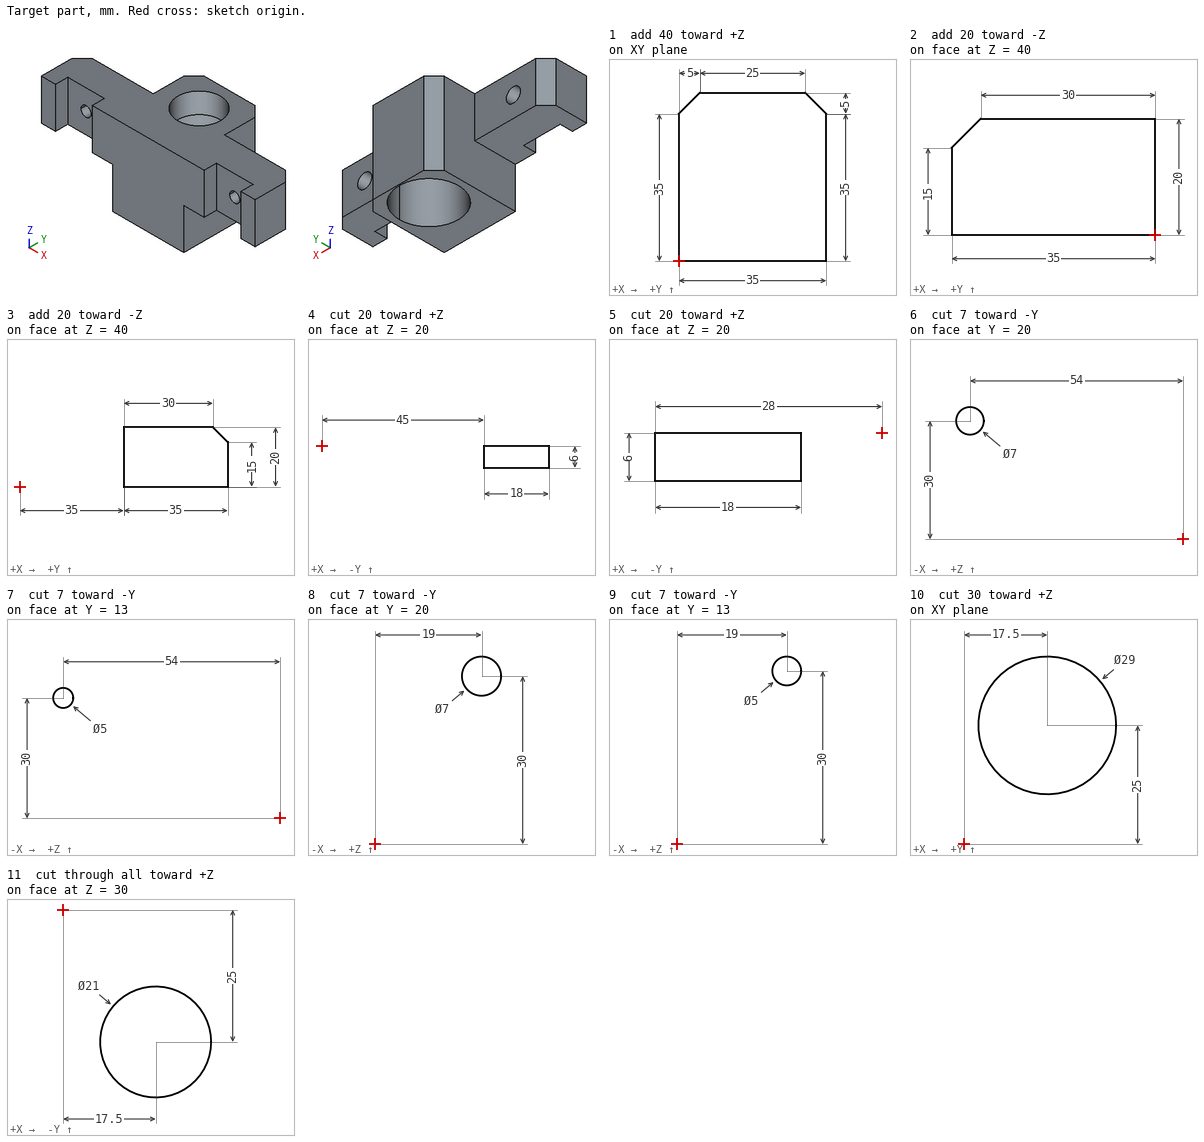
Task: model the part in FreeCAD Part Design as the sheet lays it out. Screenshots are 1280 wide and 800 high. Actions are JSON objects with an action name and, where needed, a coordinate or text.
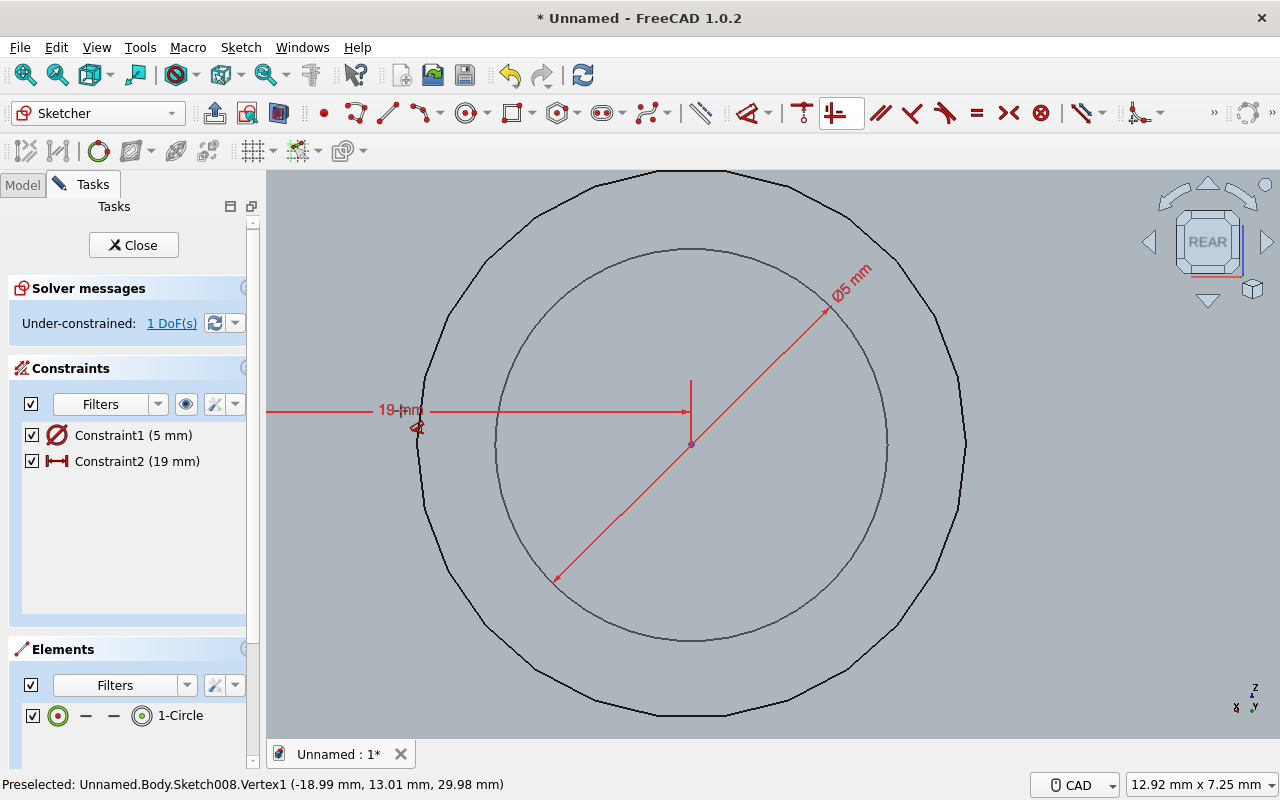
{"action": "left_click", "coordinate": [691, 445]}
{"action": "left_click", "coordinate": [725, 578]}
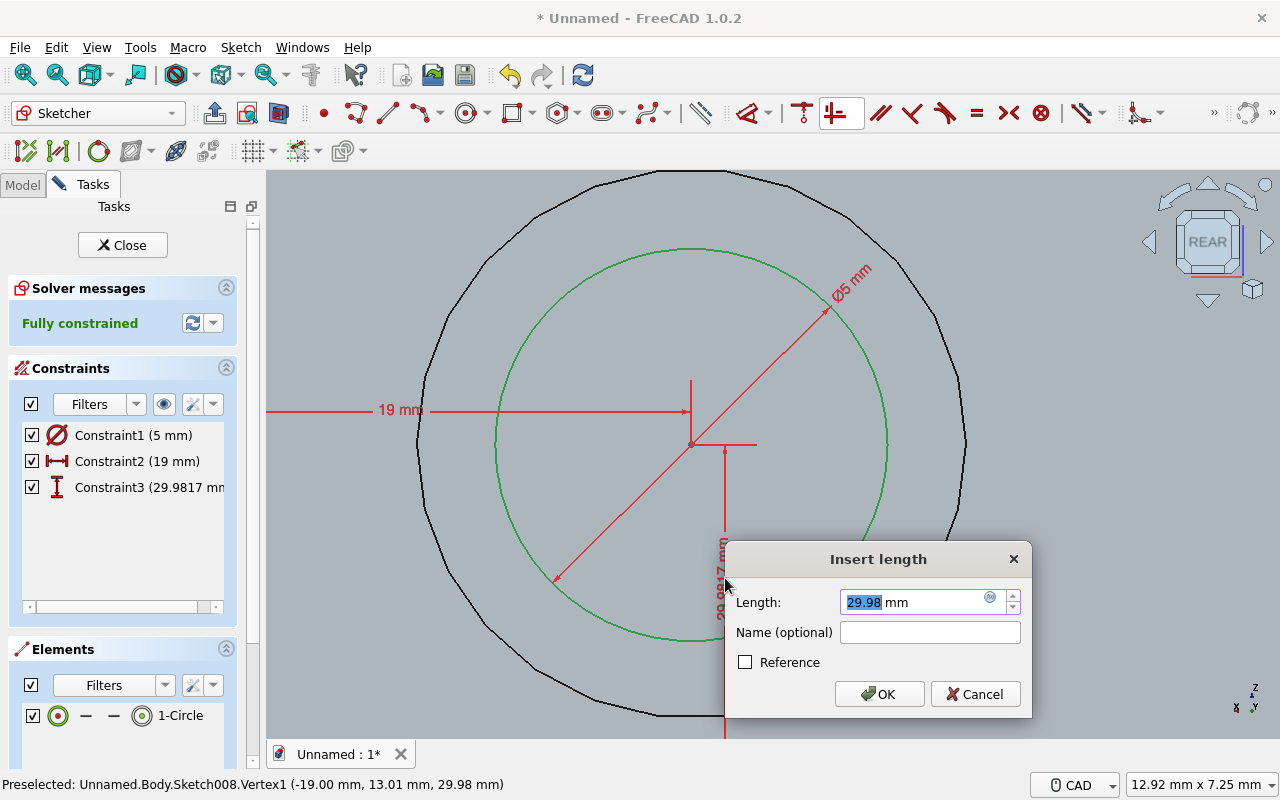
{"action": "type", "text": "30"}
{"action": "key", "text": "Return"}
{"action": "key", "text": "Escape"}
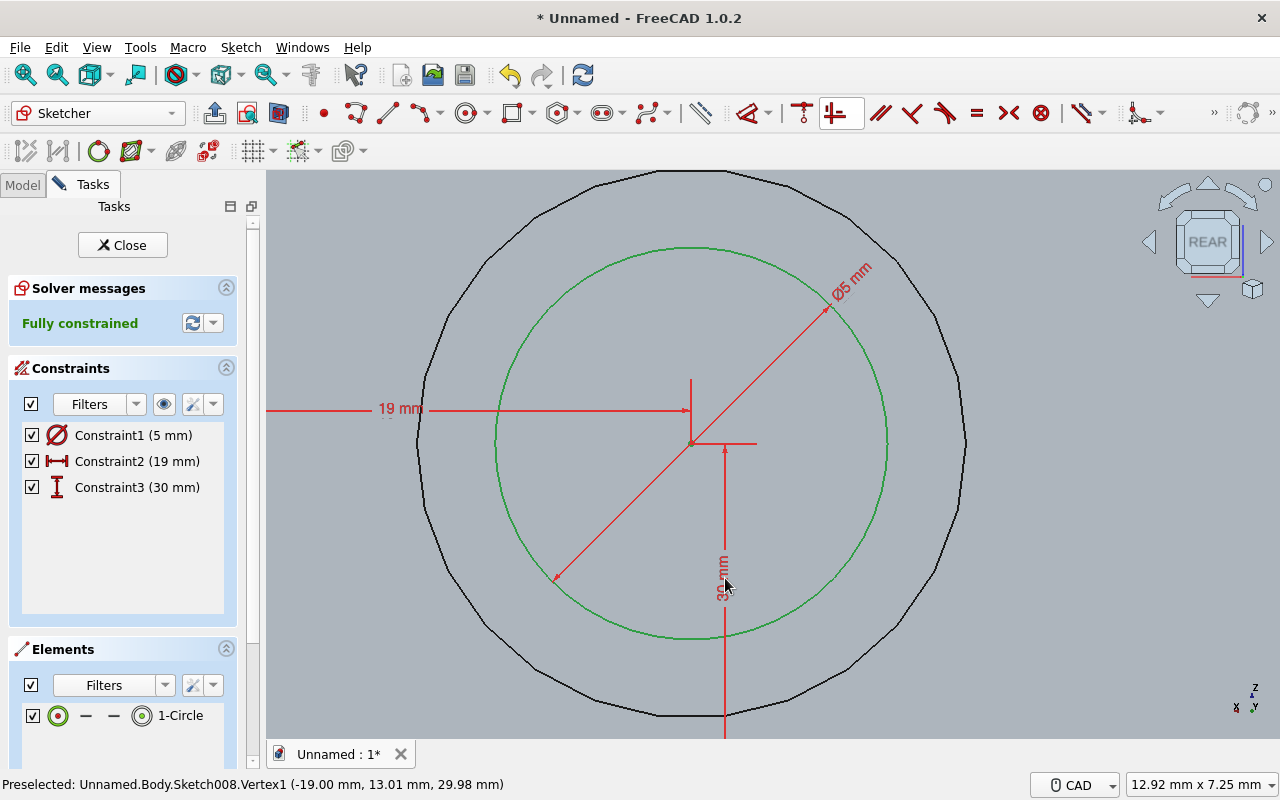
{"action": "left_click", "coordinate": [123, 245]}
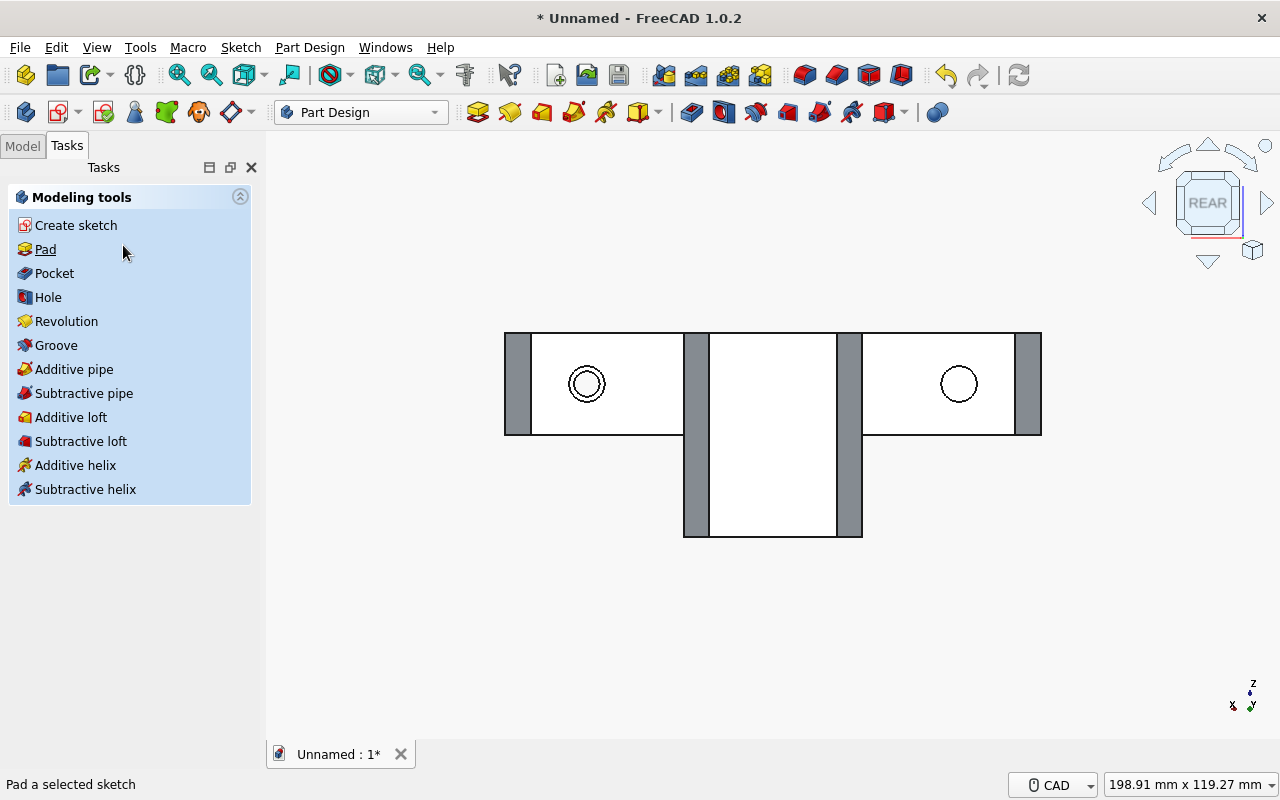
{"action": "left_click", "coordinate": [692, 112]}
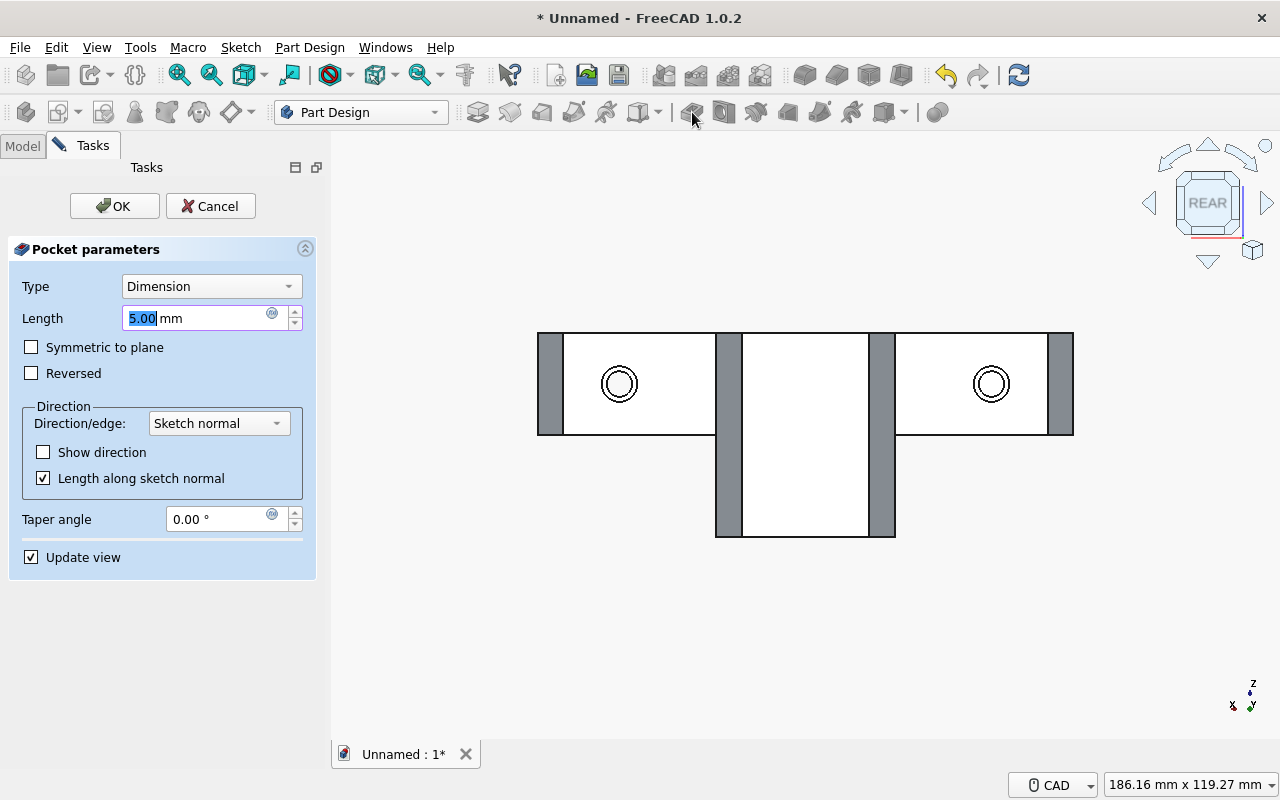
{"action": "type", "text": "7"}
{"action": "key", "text": "Tab"}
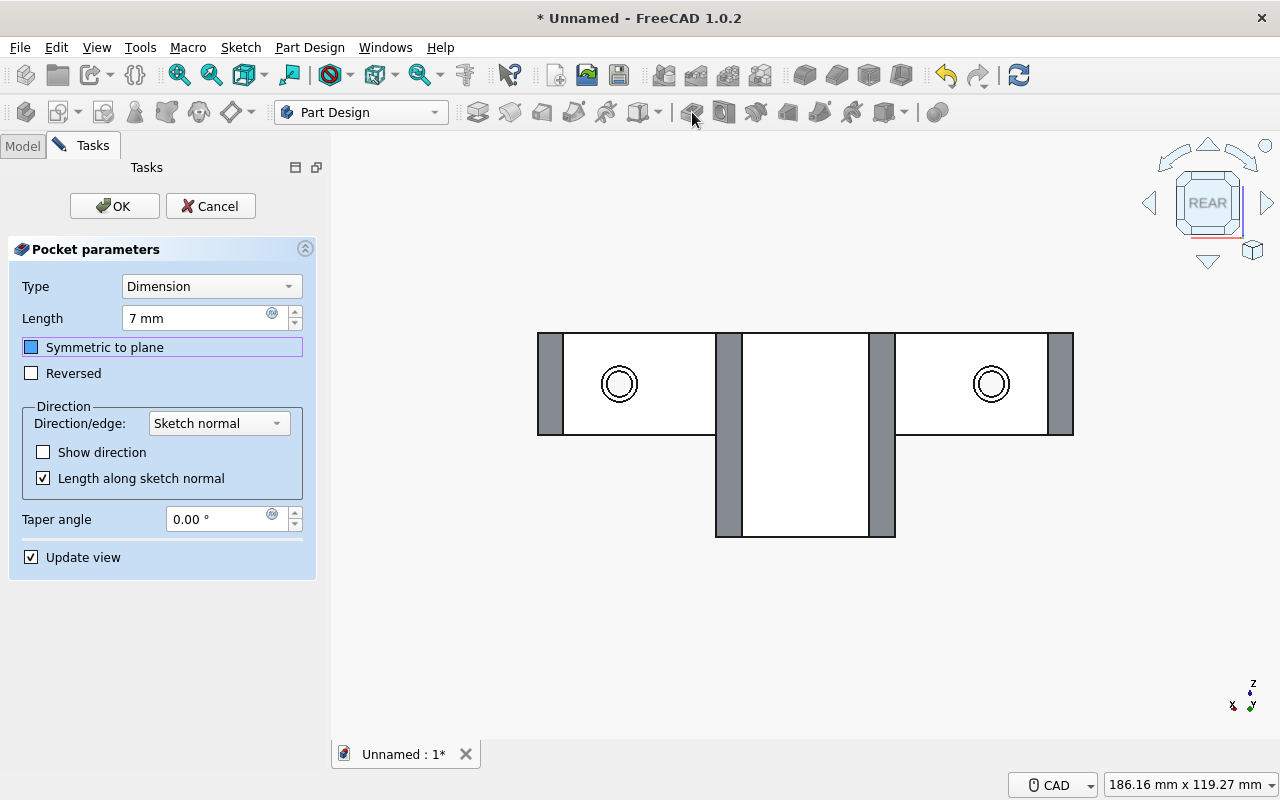
{"action": "left_click", "coordinate": [115, 206]}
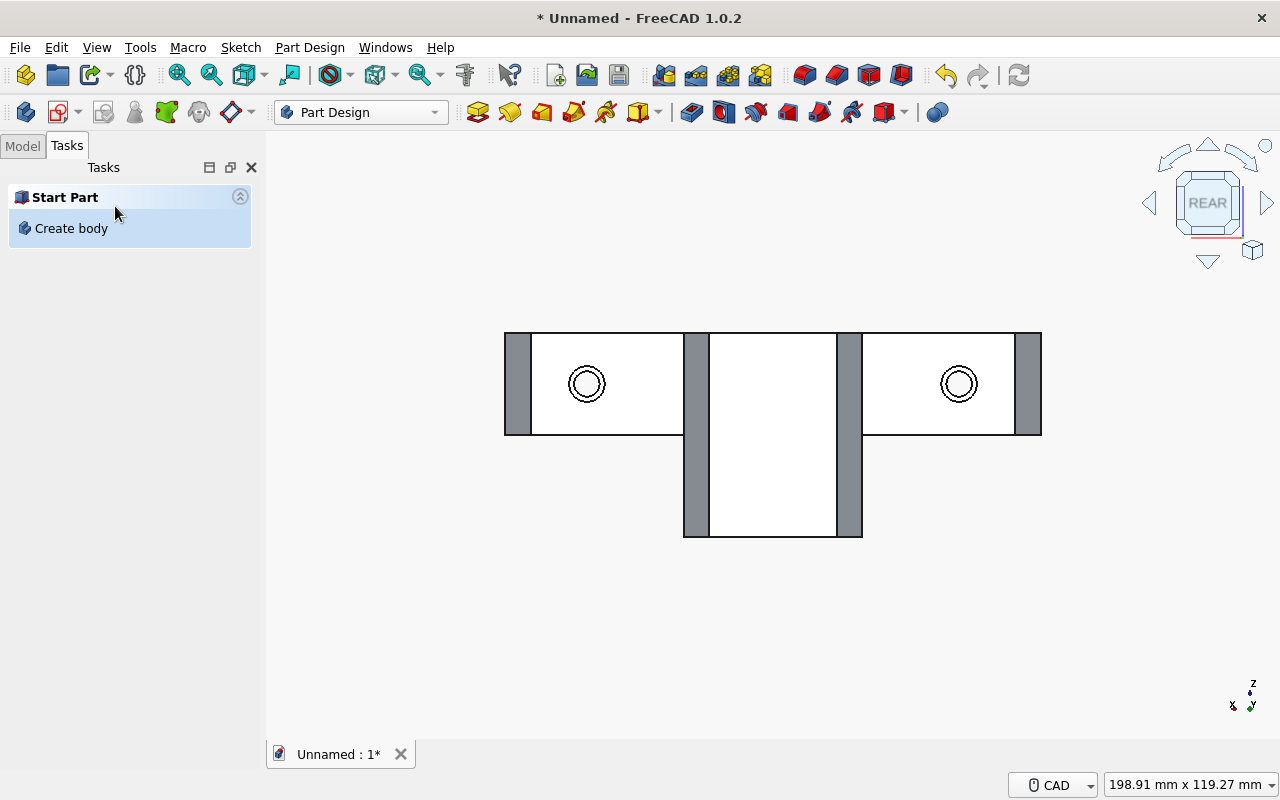
{"action": "left_click", "coordinate": [58, 112]}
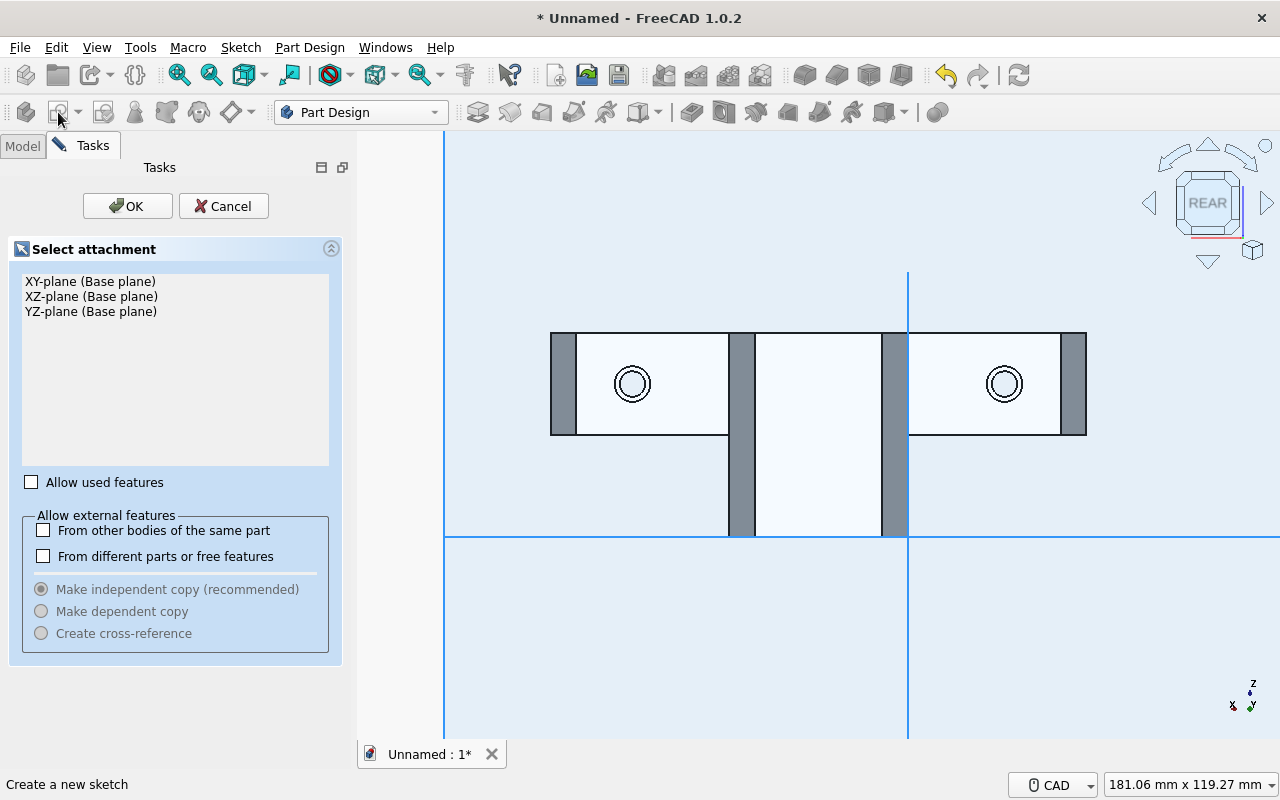
{"action": "left_click", "coordinate": [82, 282]}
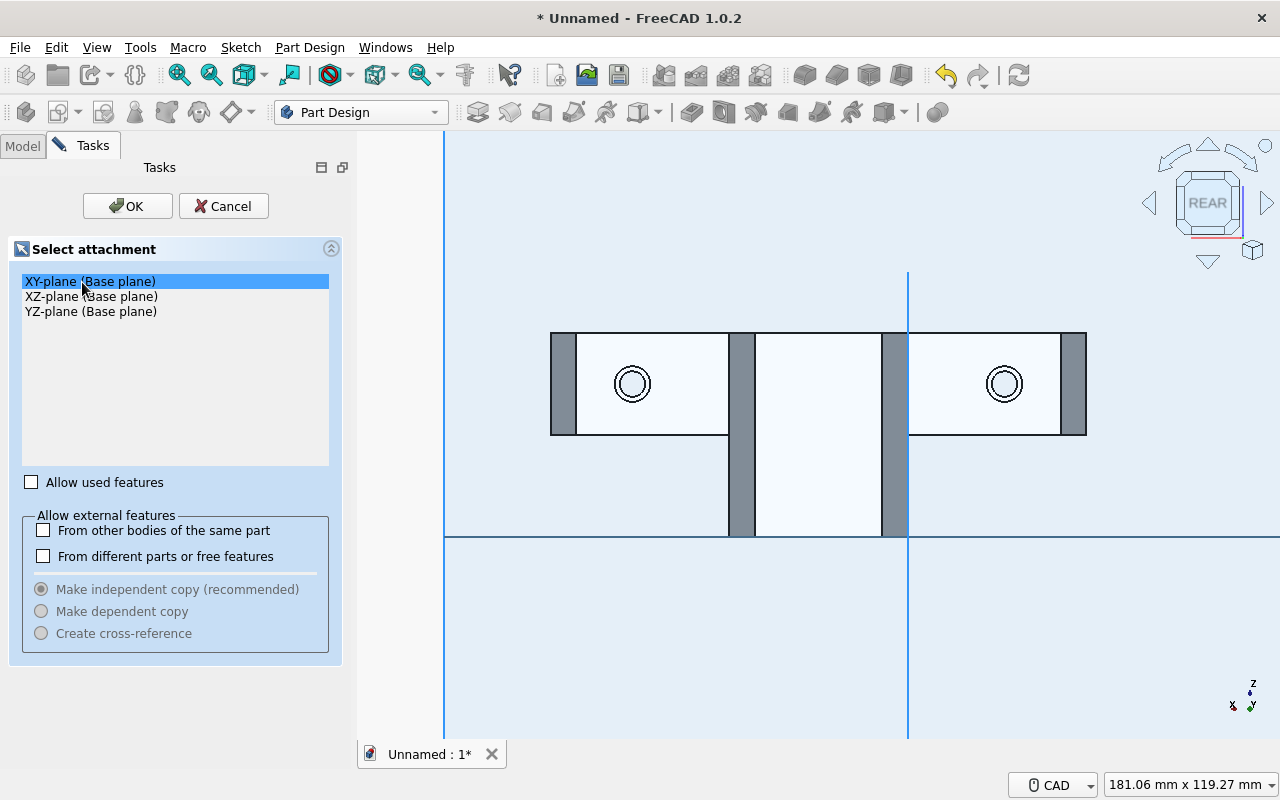
{"action": "left_click", "coordinate": [128, 206]}